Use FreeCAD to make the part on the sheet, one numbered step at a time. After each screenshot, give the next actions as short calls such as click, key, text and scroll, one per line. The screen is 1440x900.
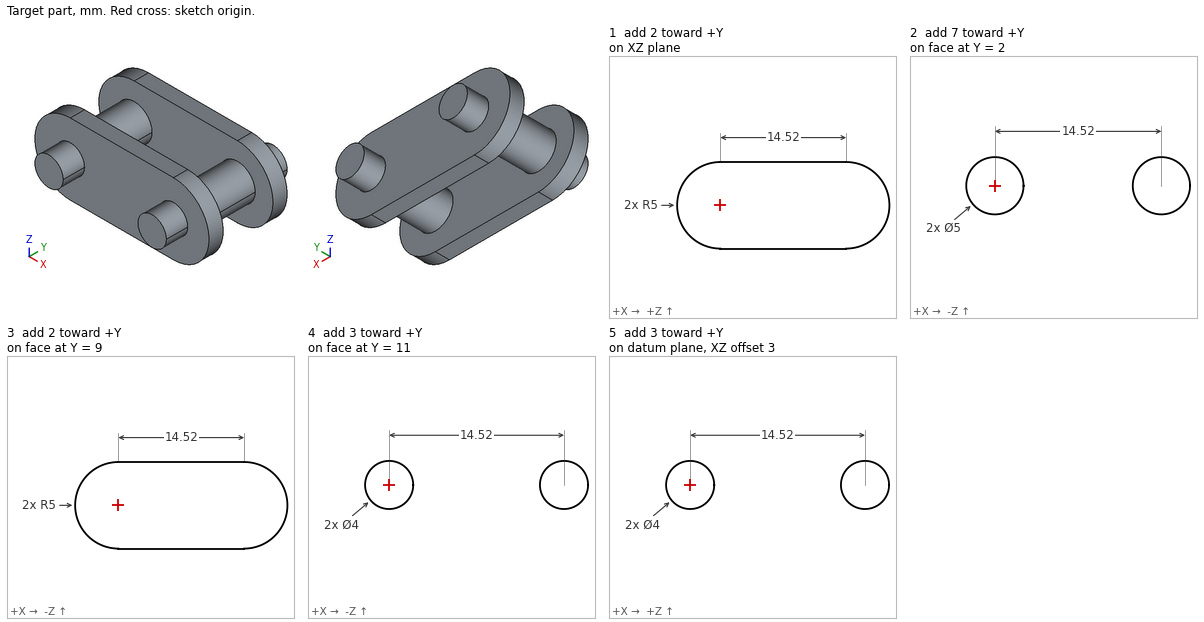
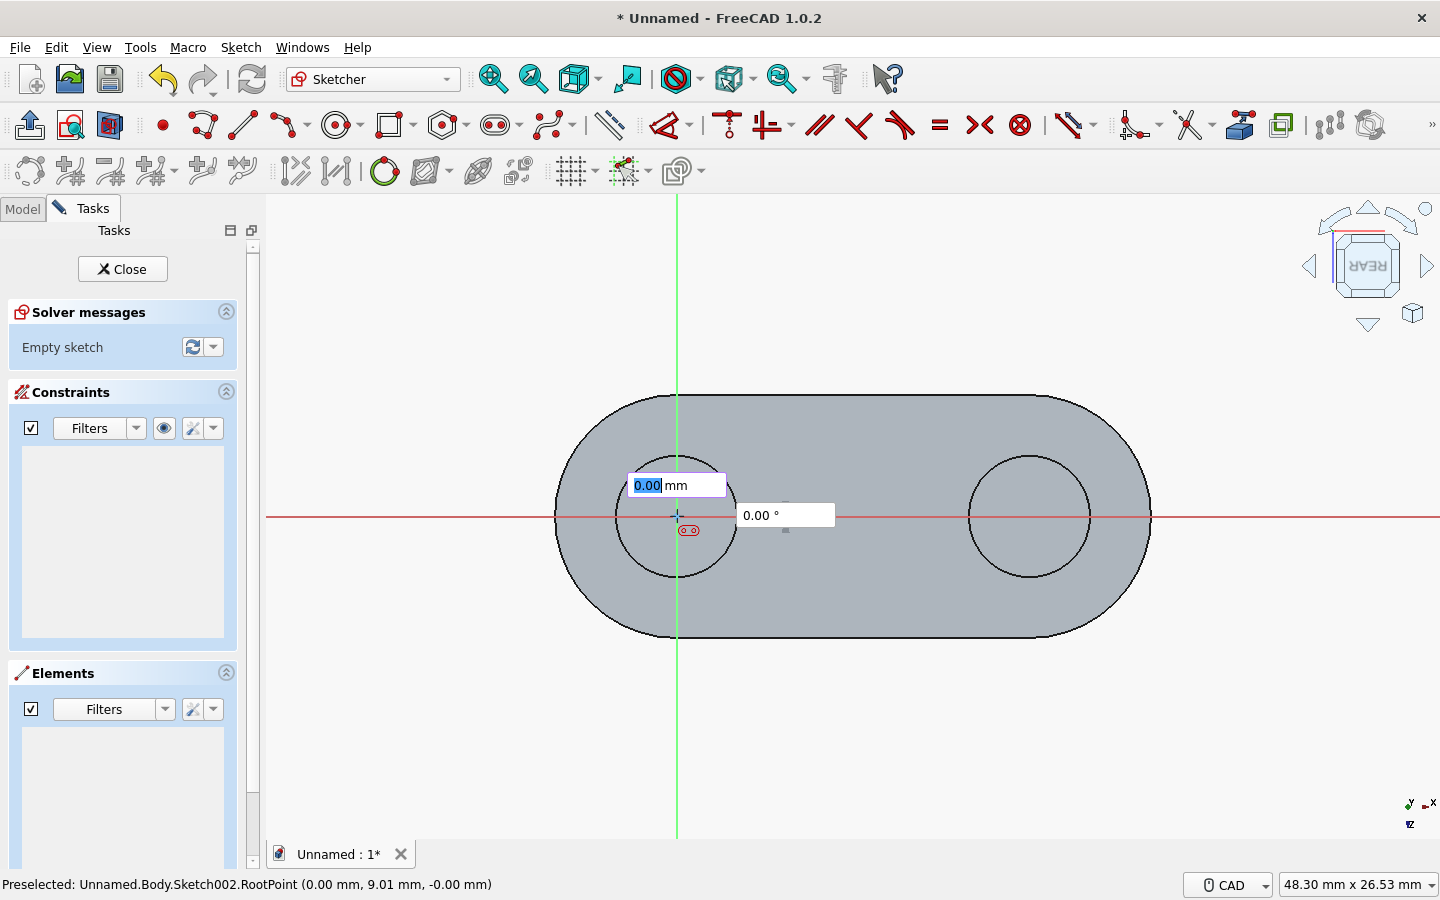
click(1029, 507)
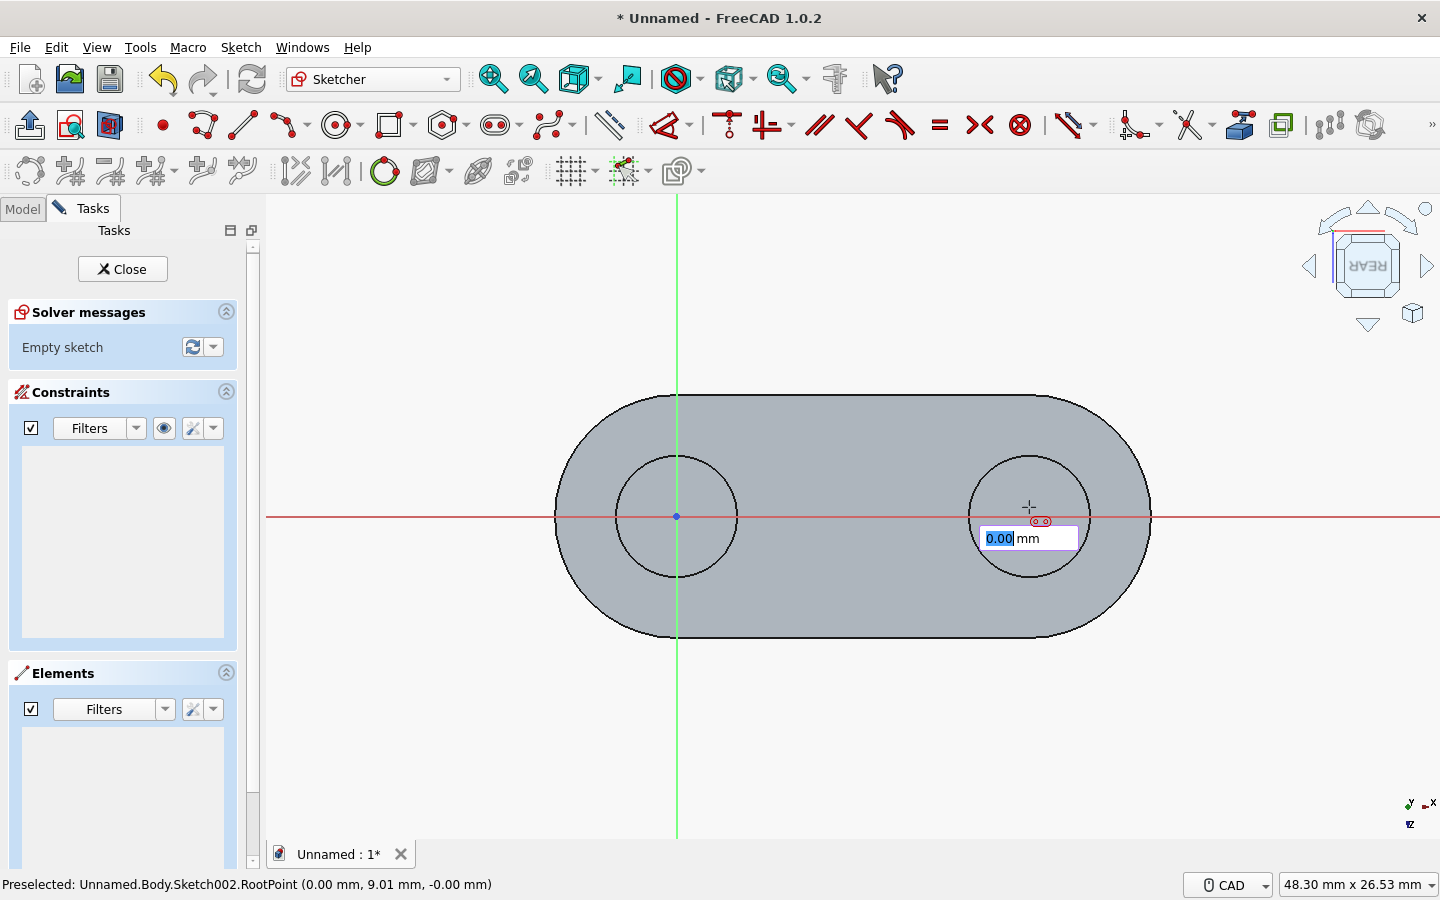
click(853, 395)
key(Escape)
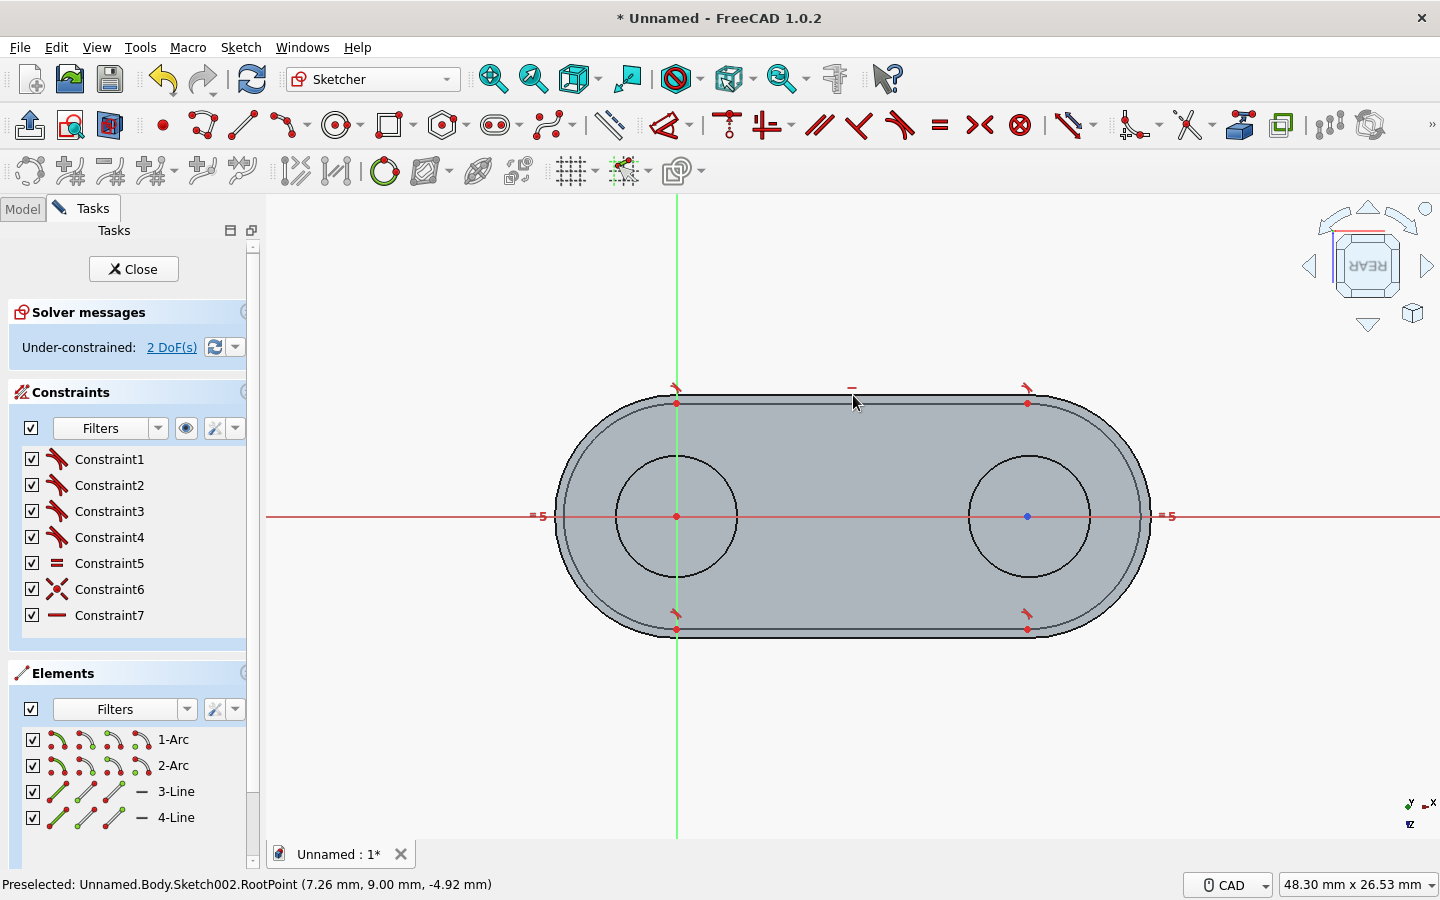
click(664, 126)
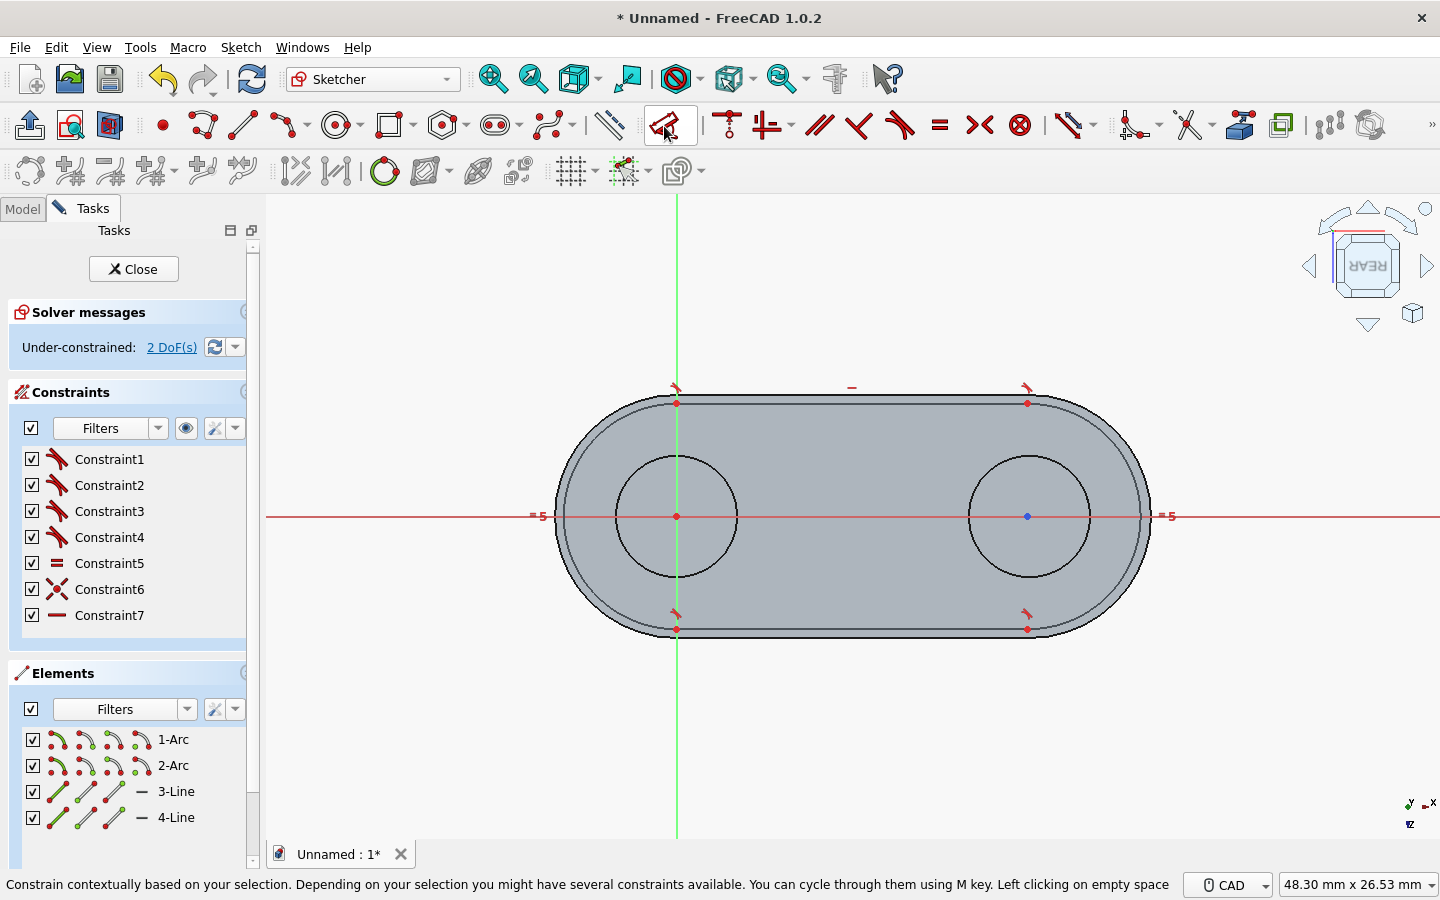
click(585, 450)
click(559, 431)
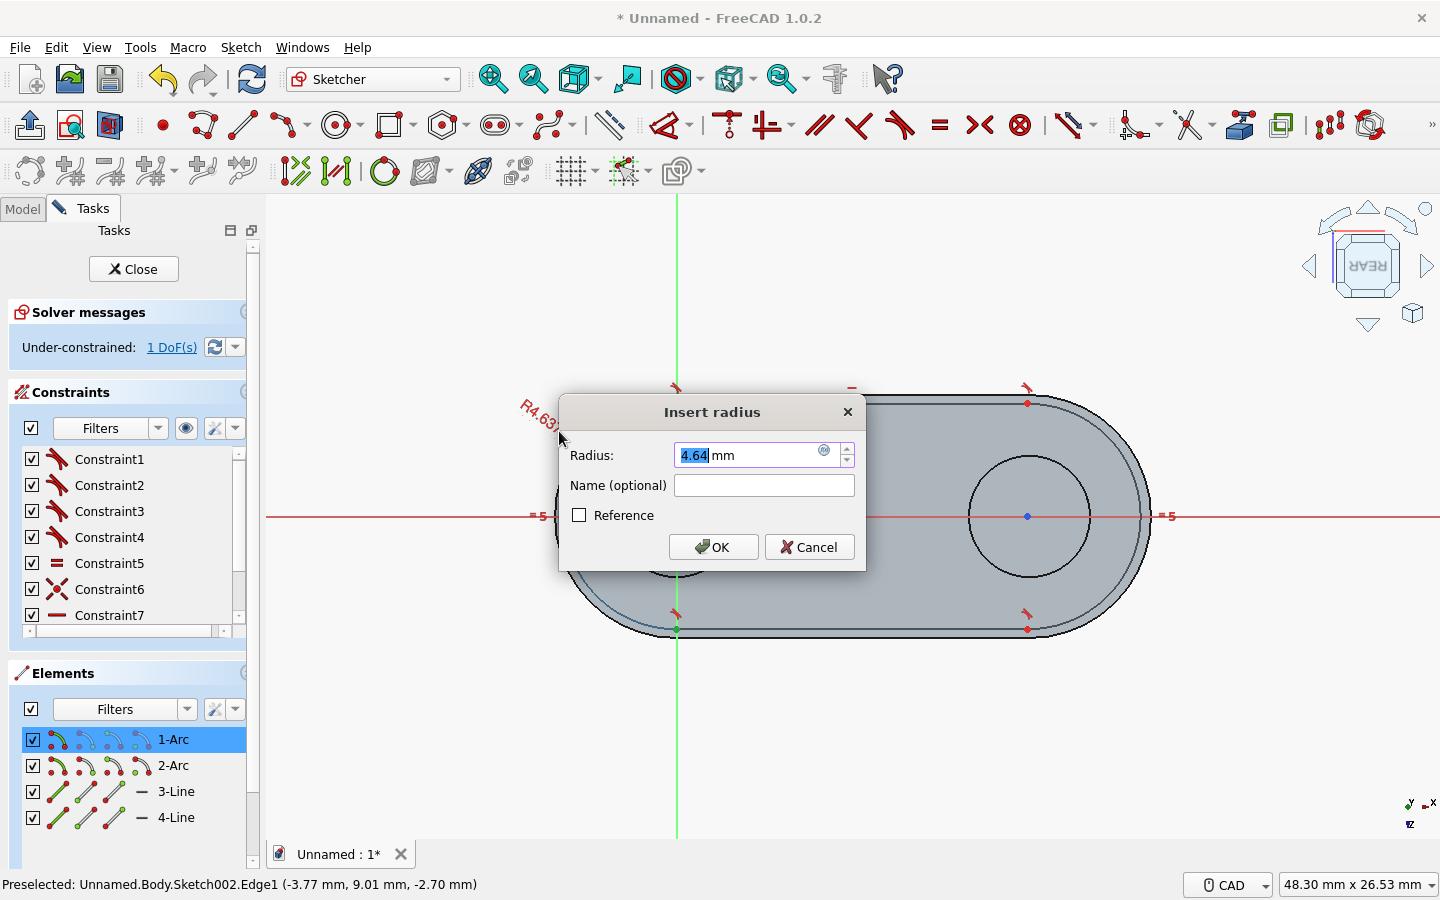
text(5)
key(Return)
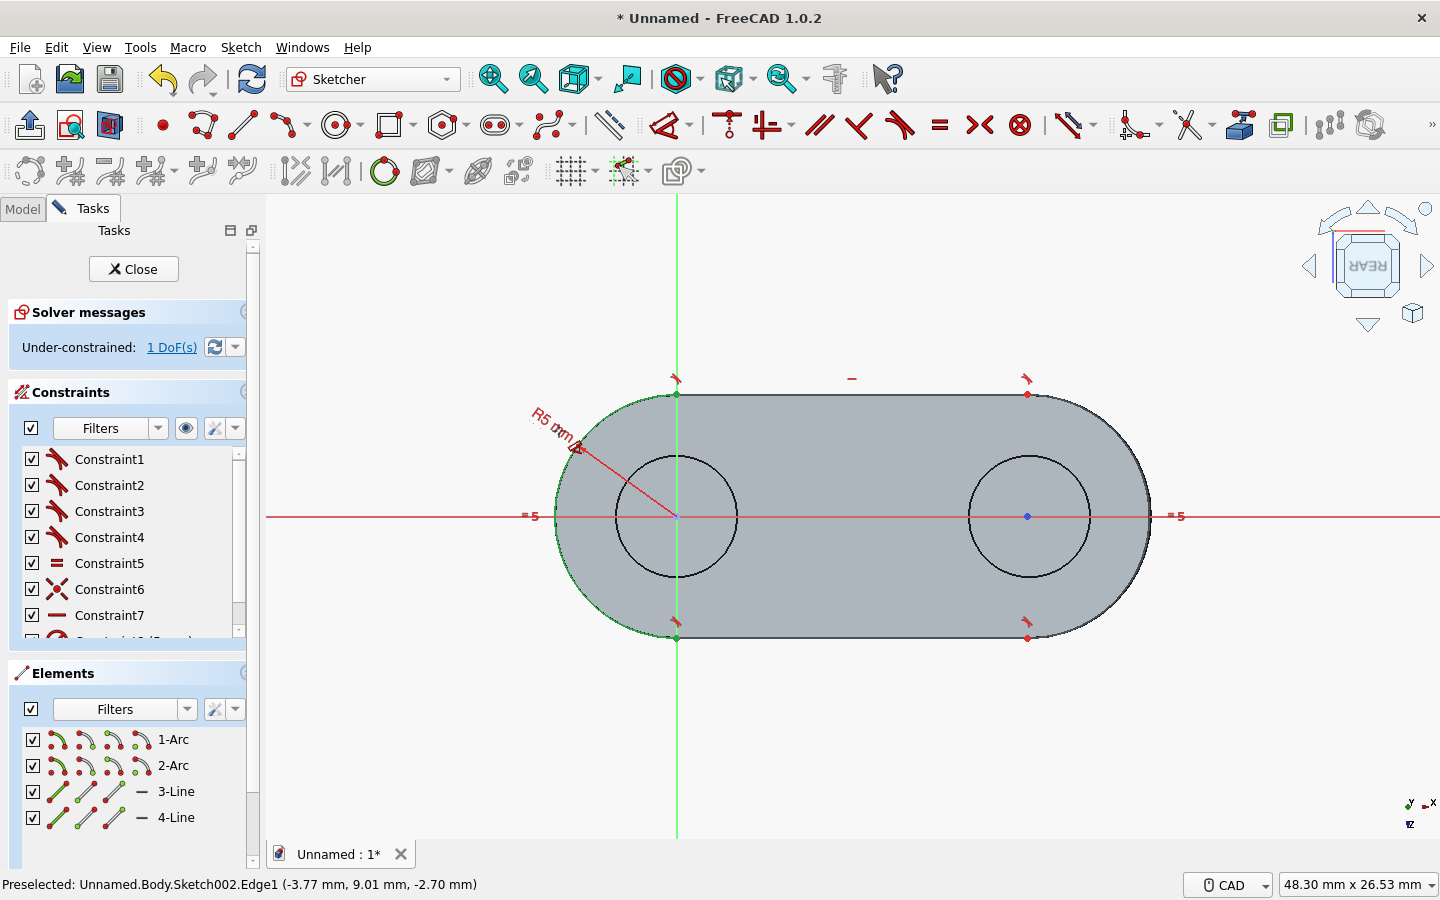
click(782, 395)
click(852, 361)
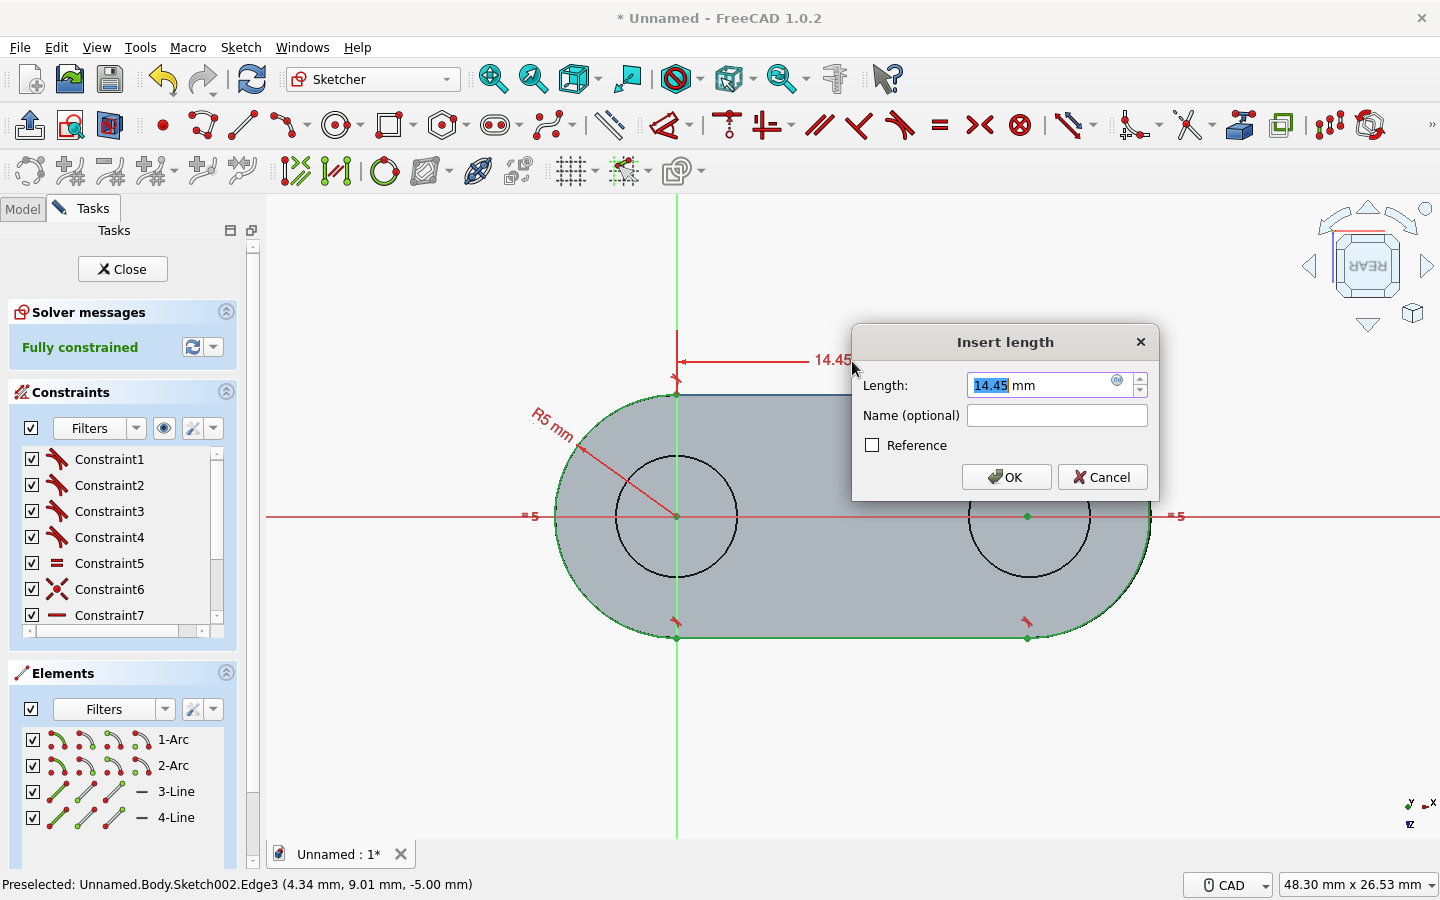
text(14.52)
key(Return)
key(Escape)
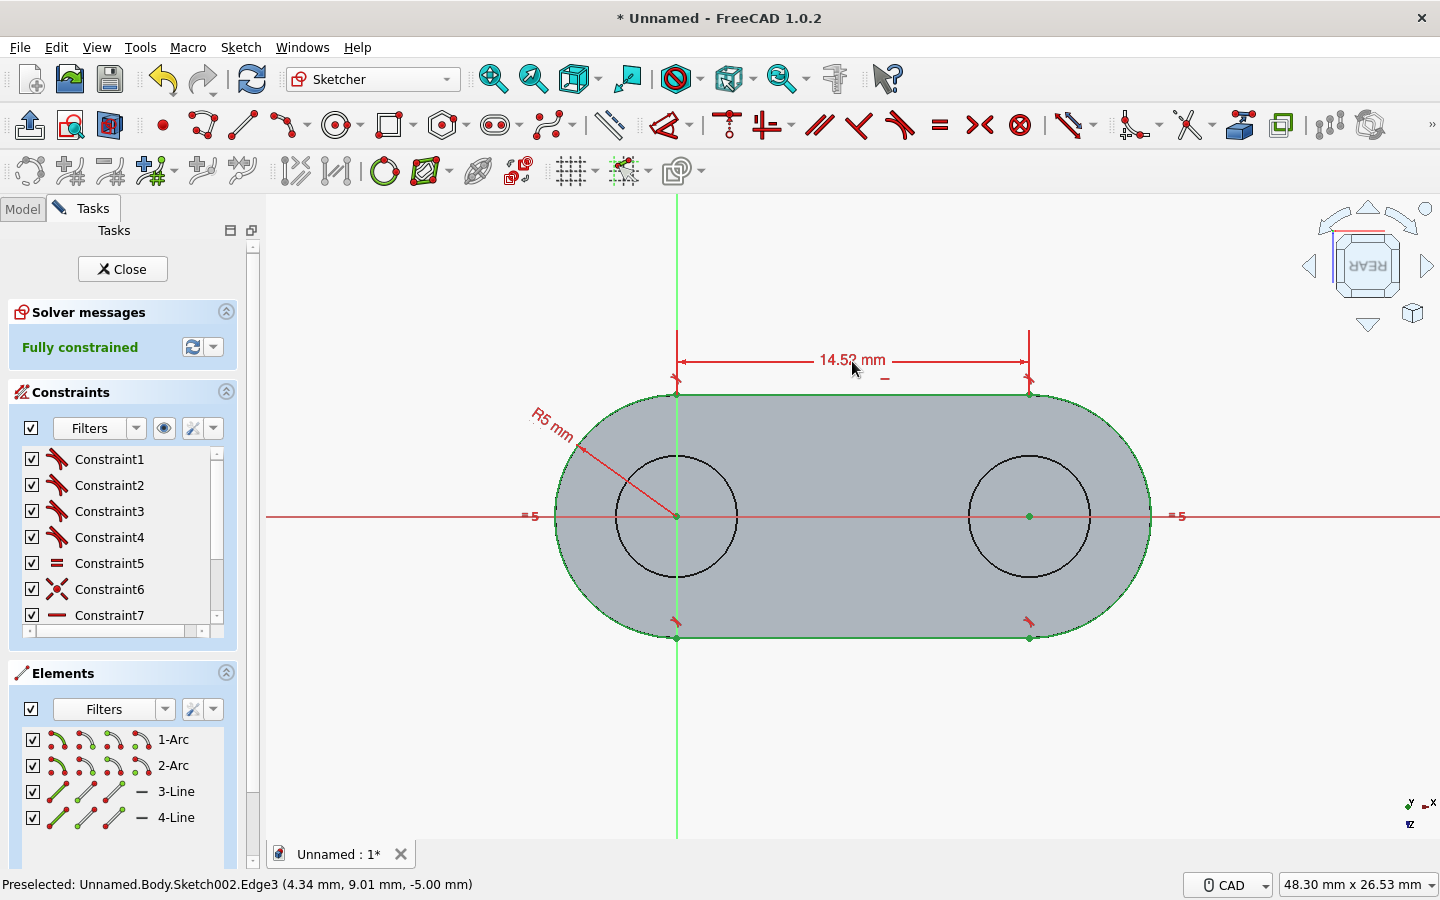
click(123, 269)